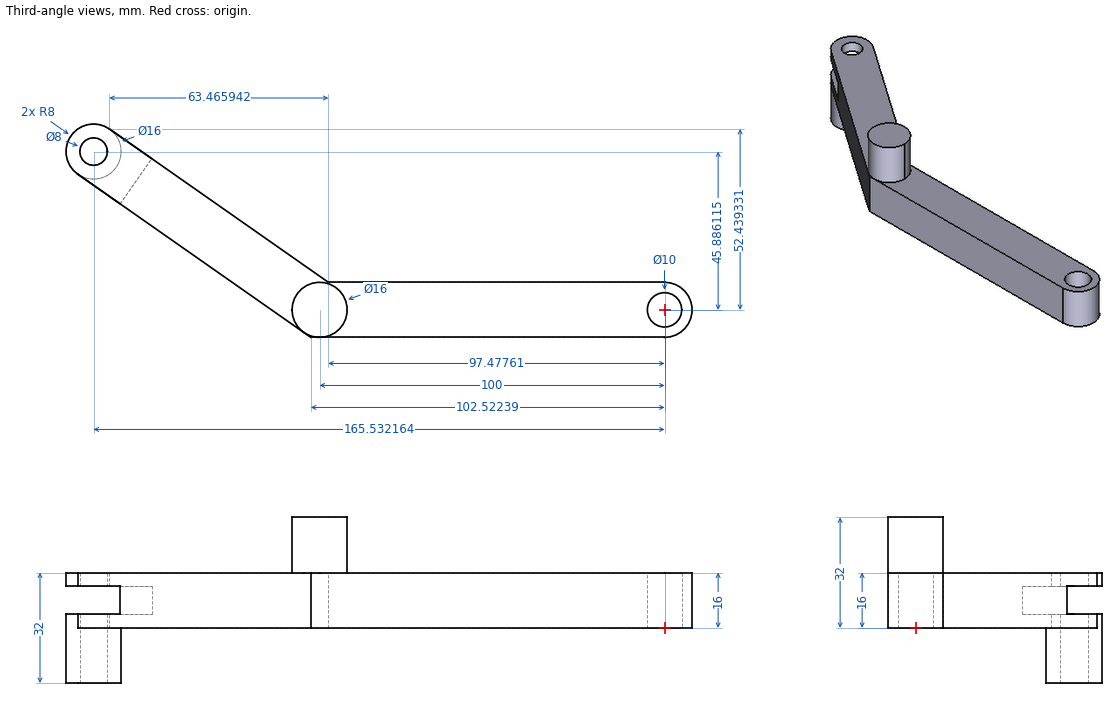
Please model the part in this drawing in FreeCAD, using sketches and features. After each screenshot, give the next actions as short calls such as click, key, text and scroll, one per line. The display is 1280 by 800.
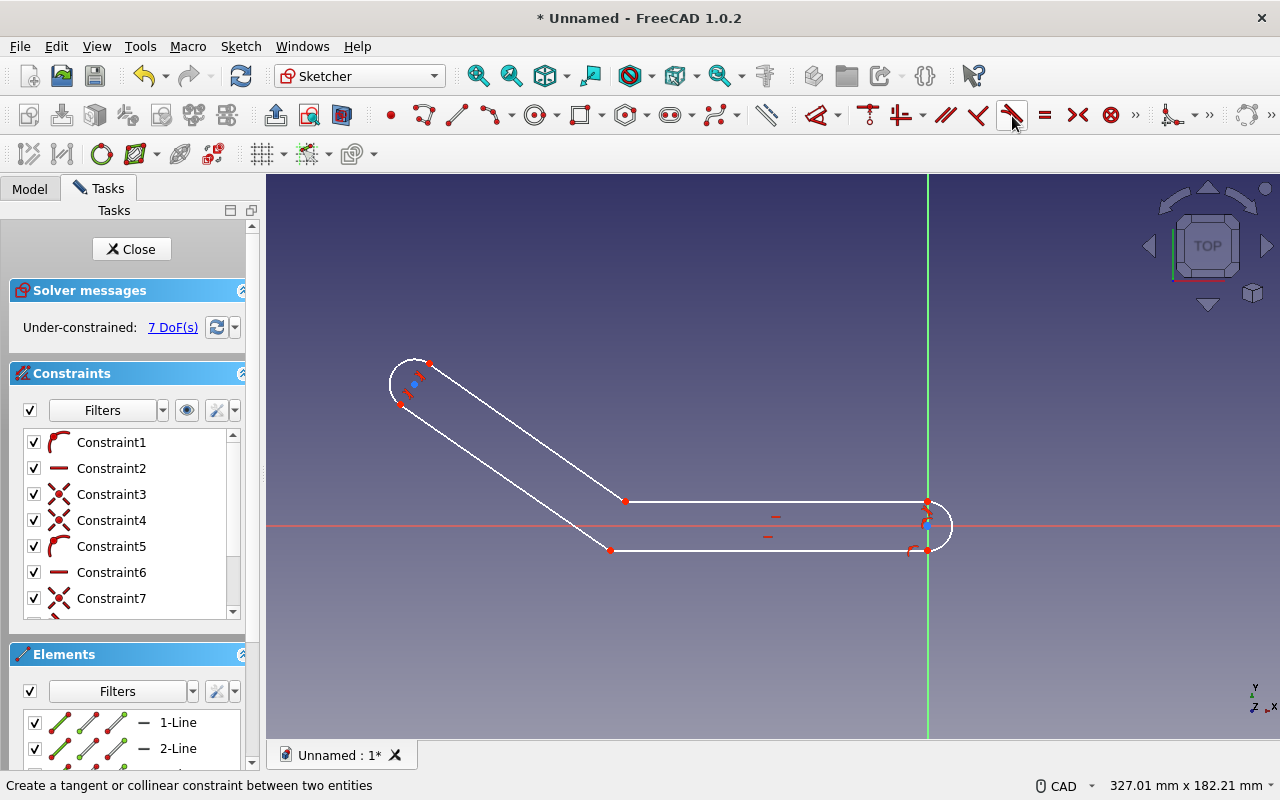
click(406, 361)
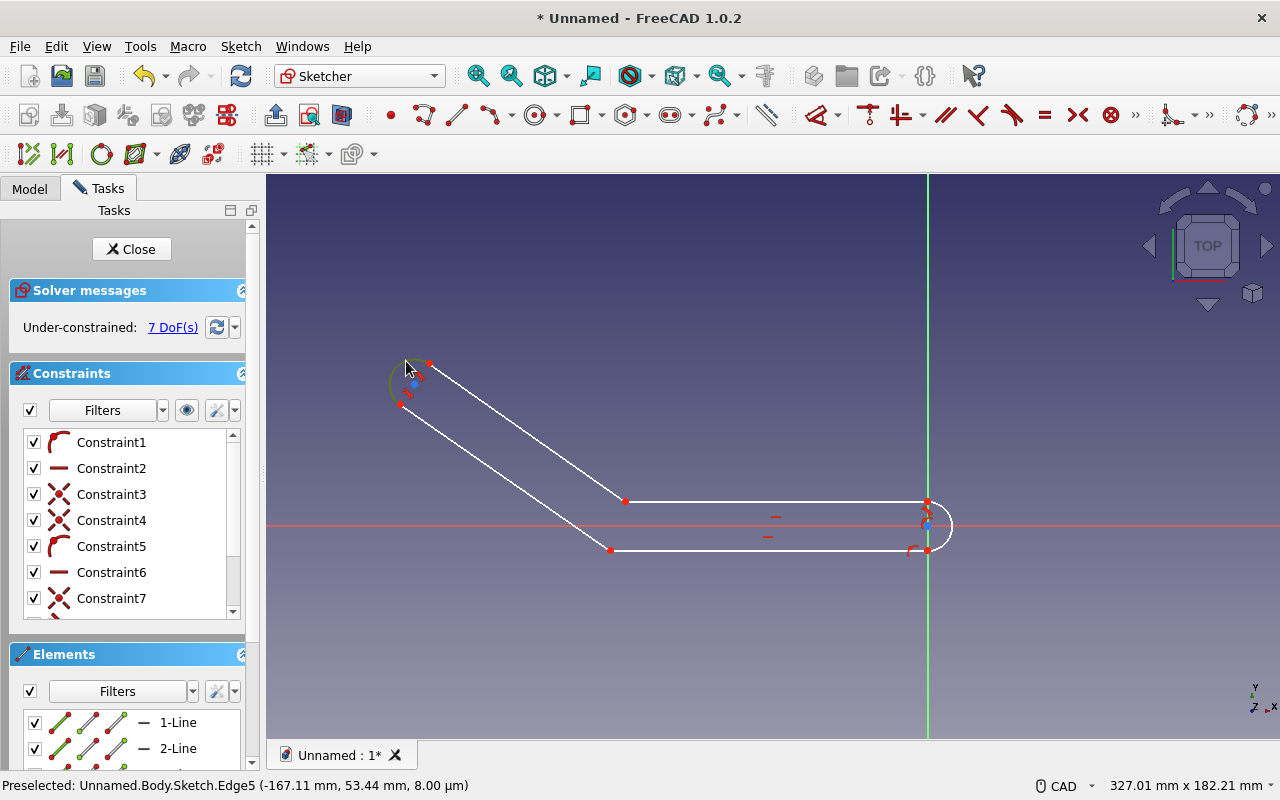
click(948, 541)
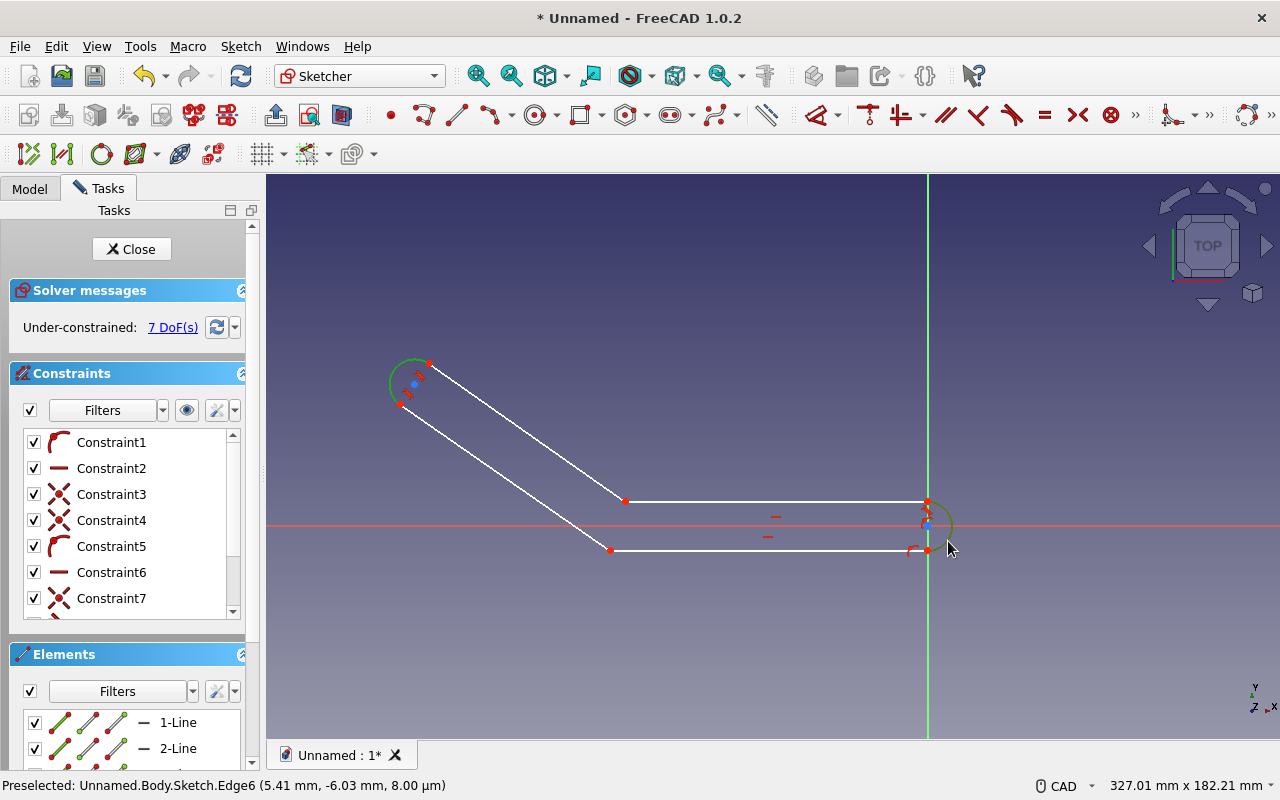
click(1045, 116)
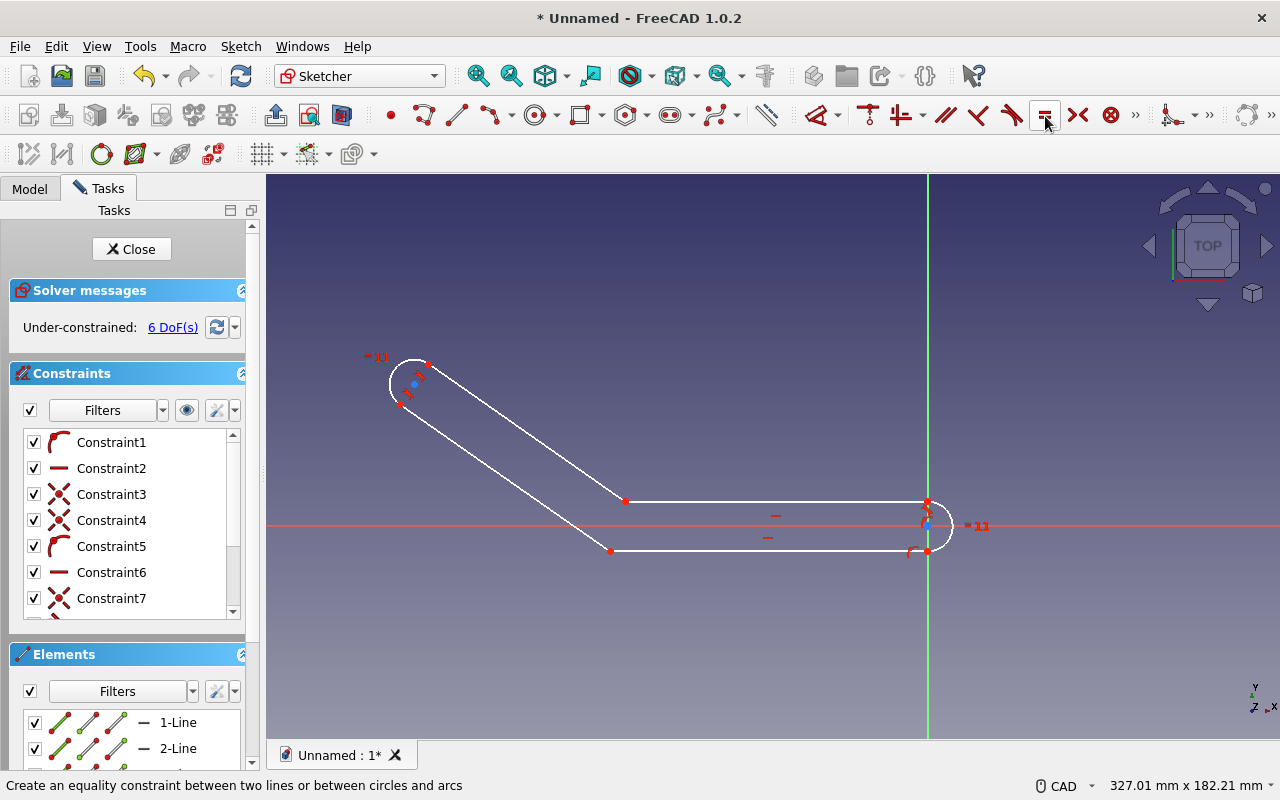
click(928, 526)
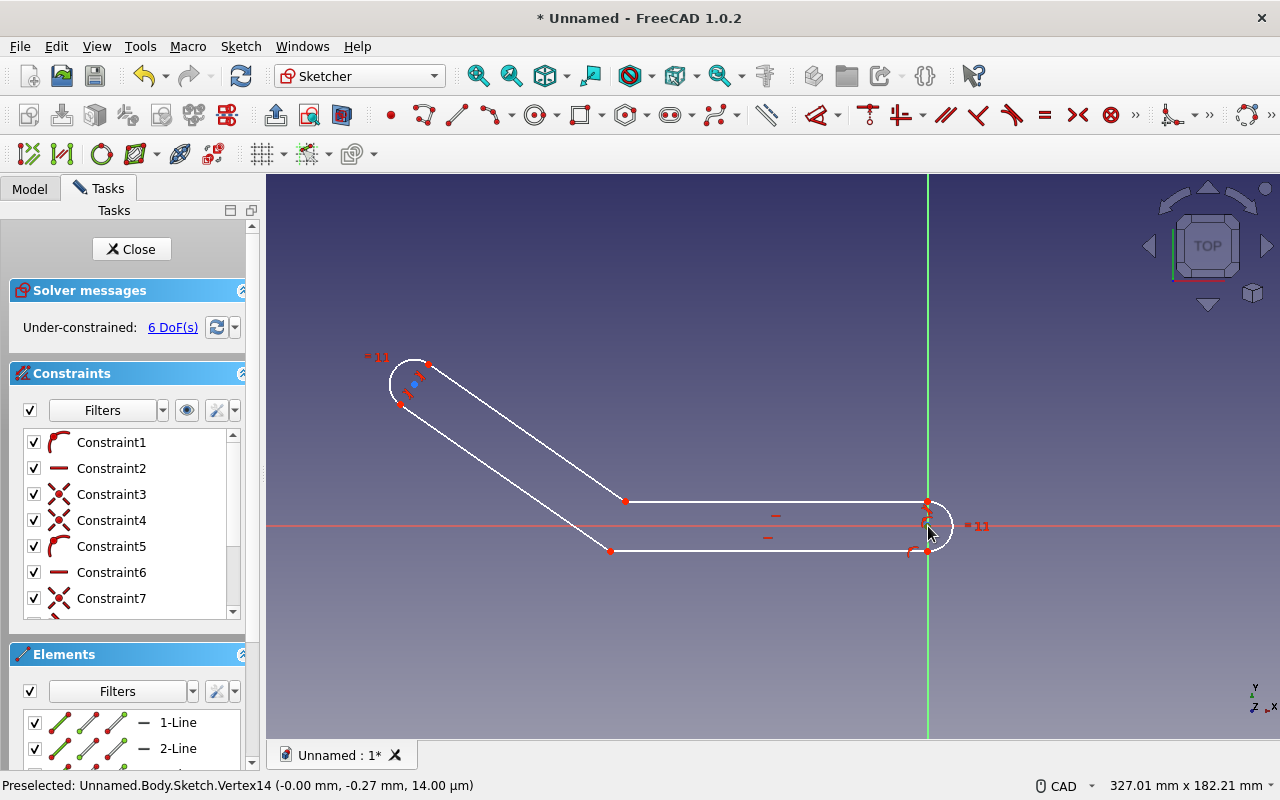
click(353, 526)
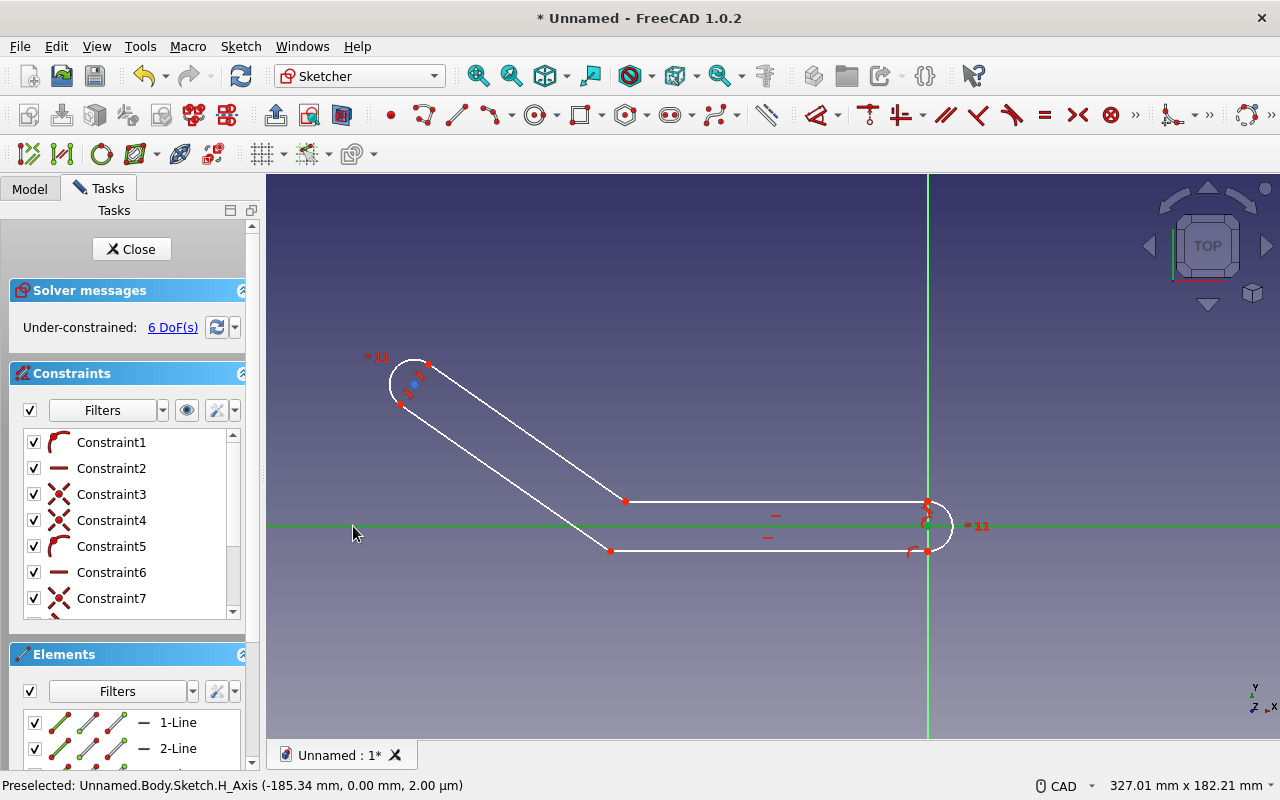
click(868, 116)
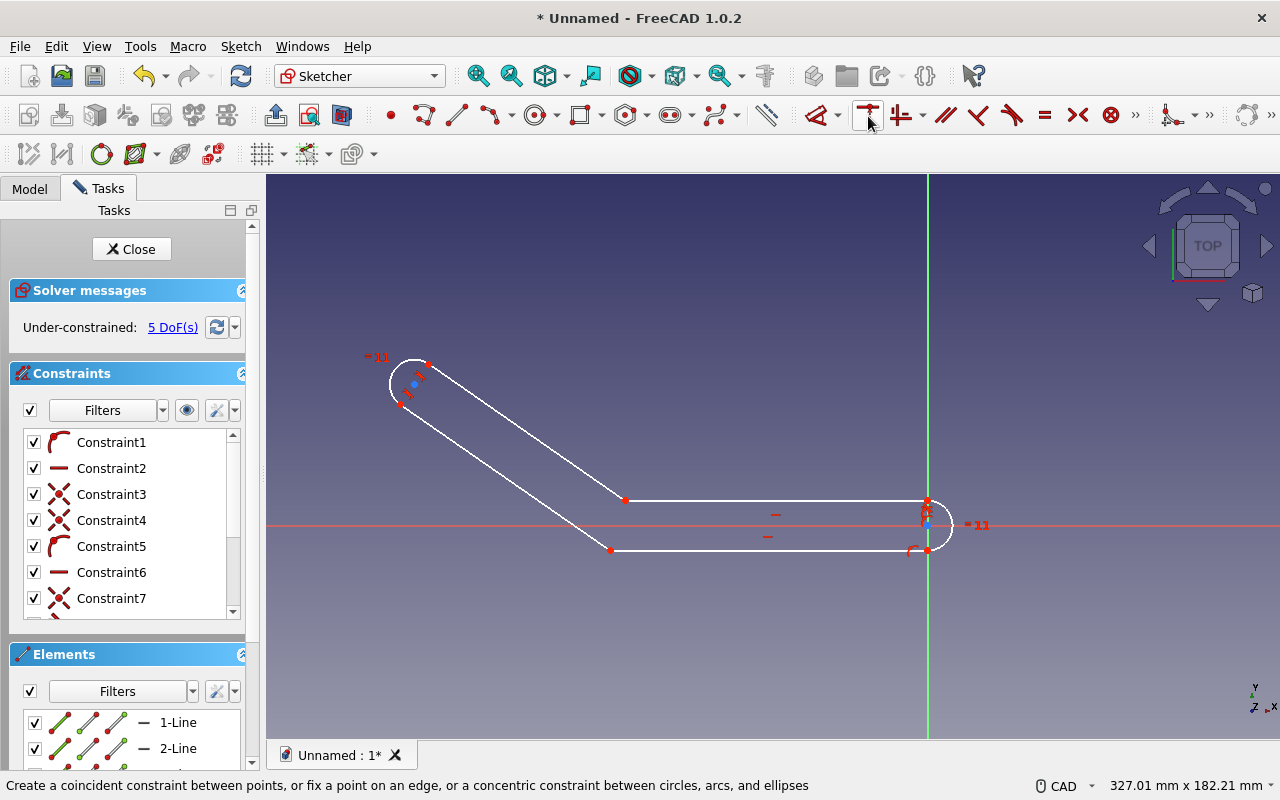
key(d)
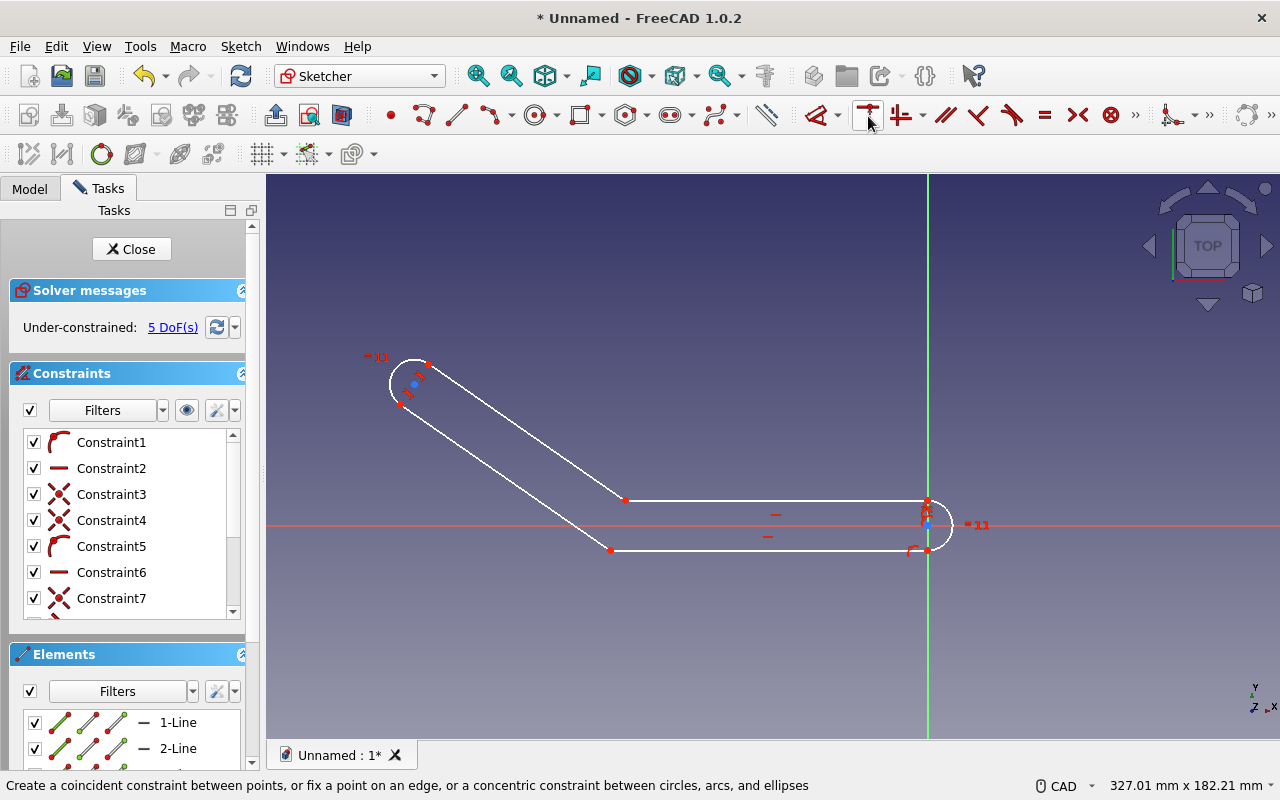
scroll(407, 361, up, 3)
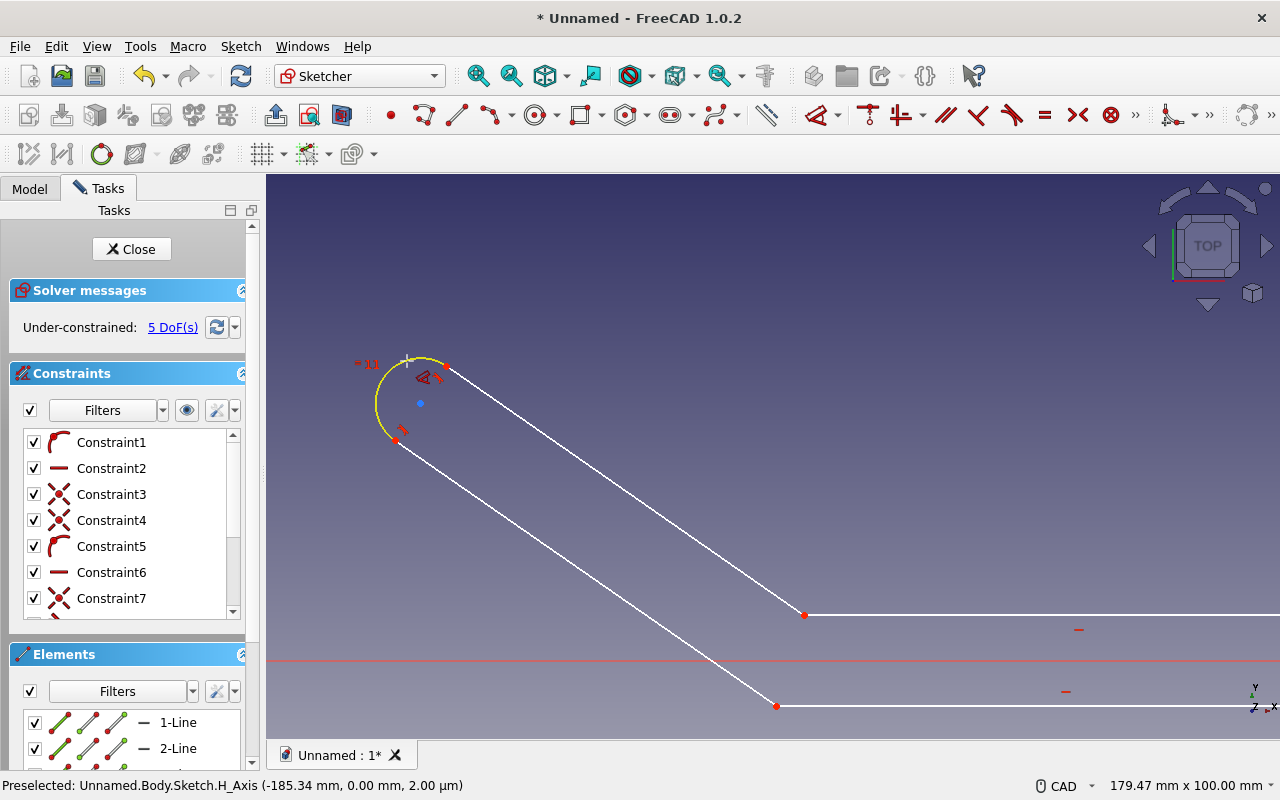
click(406, 361)
click(395, 331)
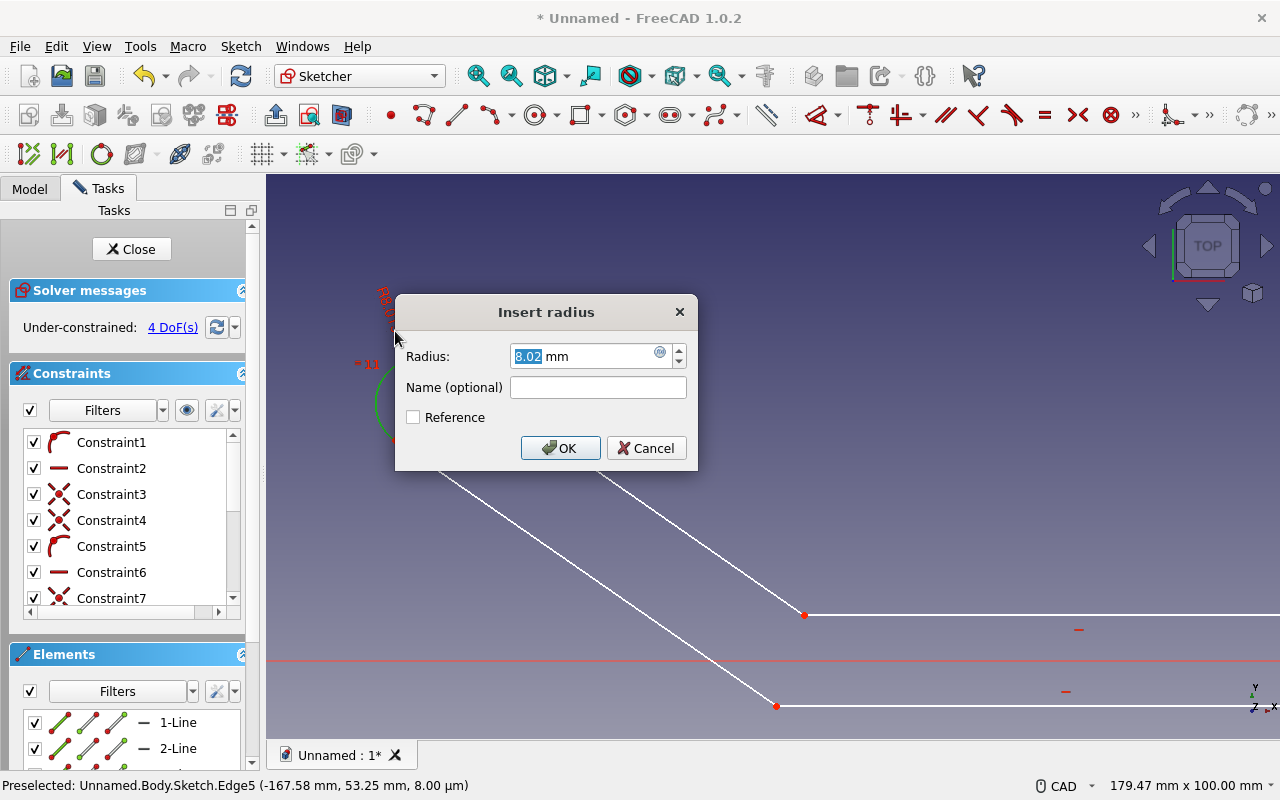
text(8)
key(Return)